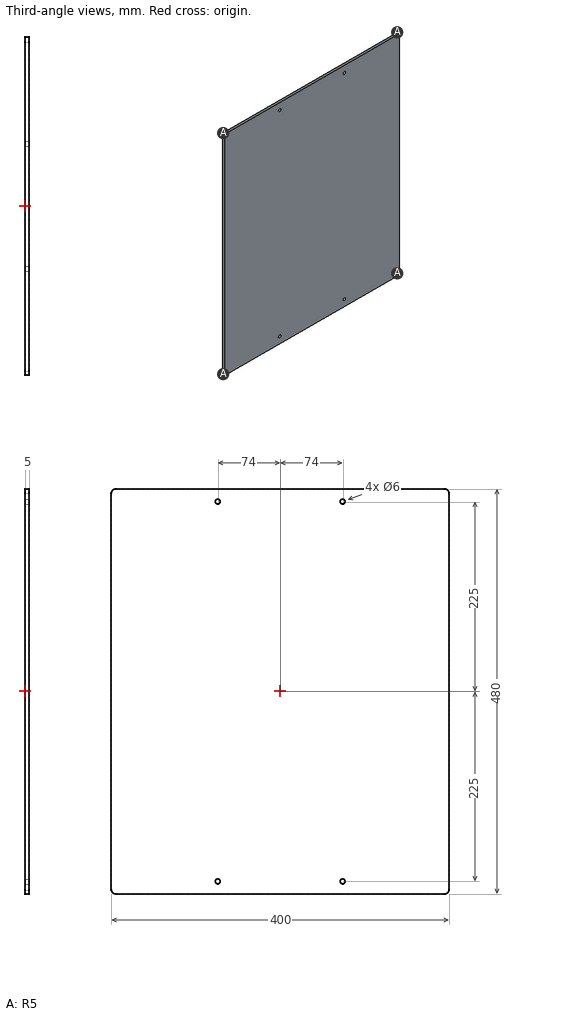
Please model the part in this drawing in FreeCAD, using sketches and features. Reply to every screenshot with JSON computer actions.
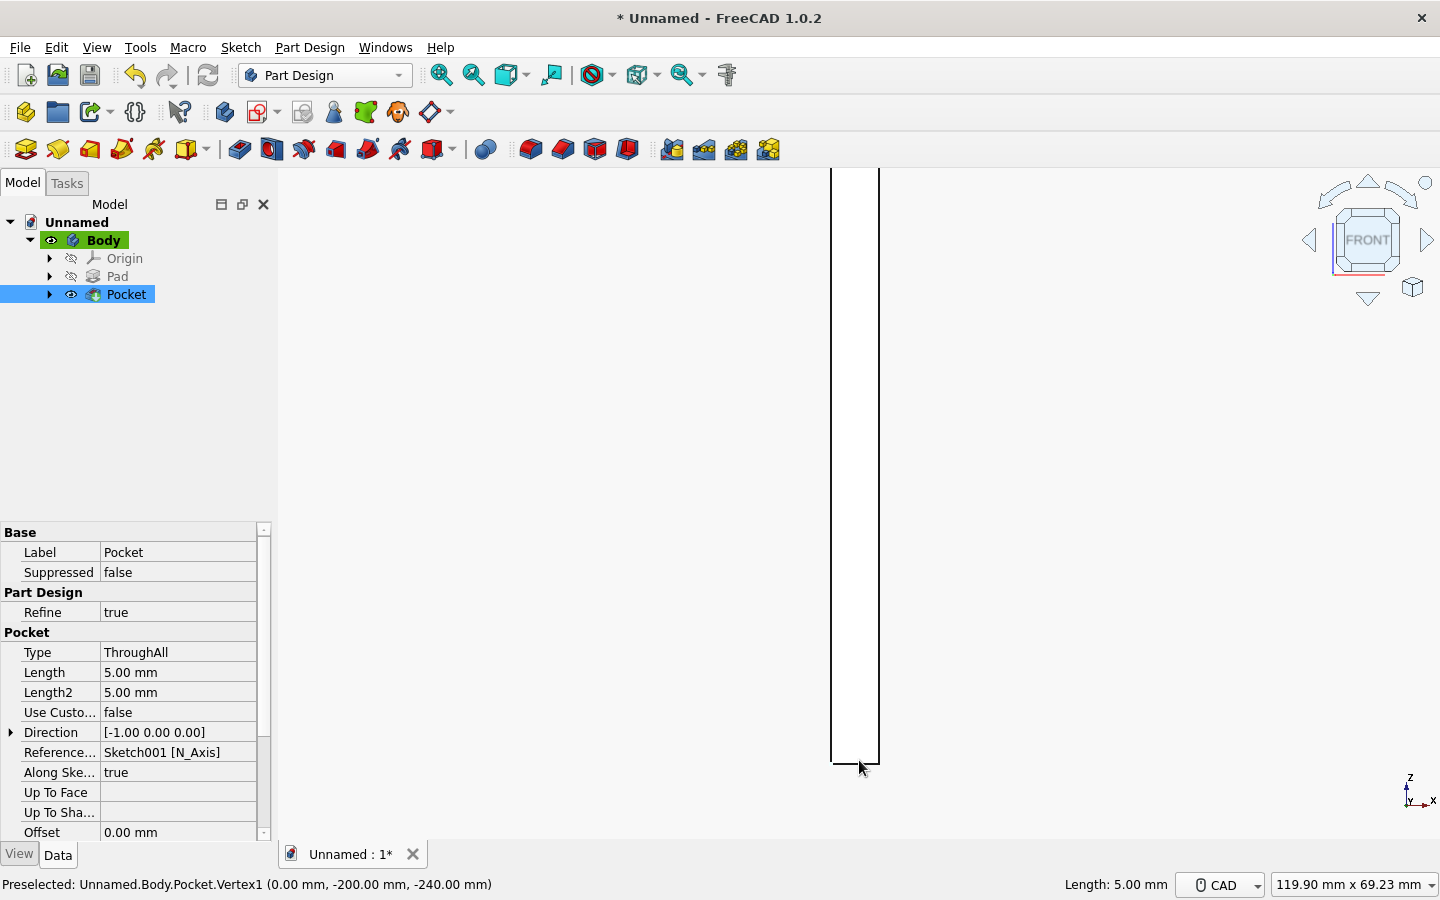
{"action": "left_click", "coordinate": [855, 763], "text": "ctrl"}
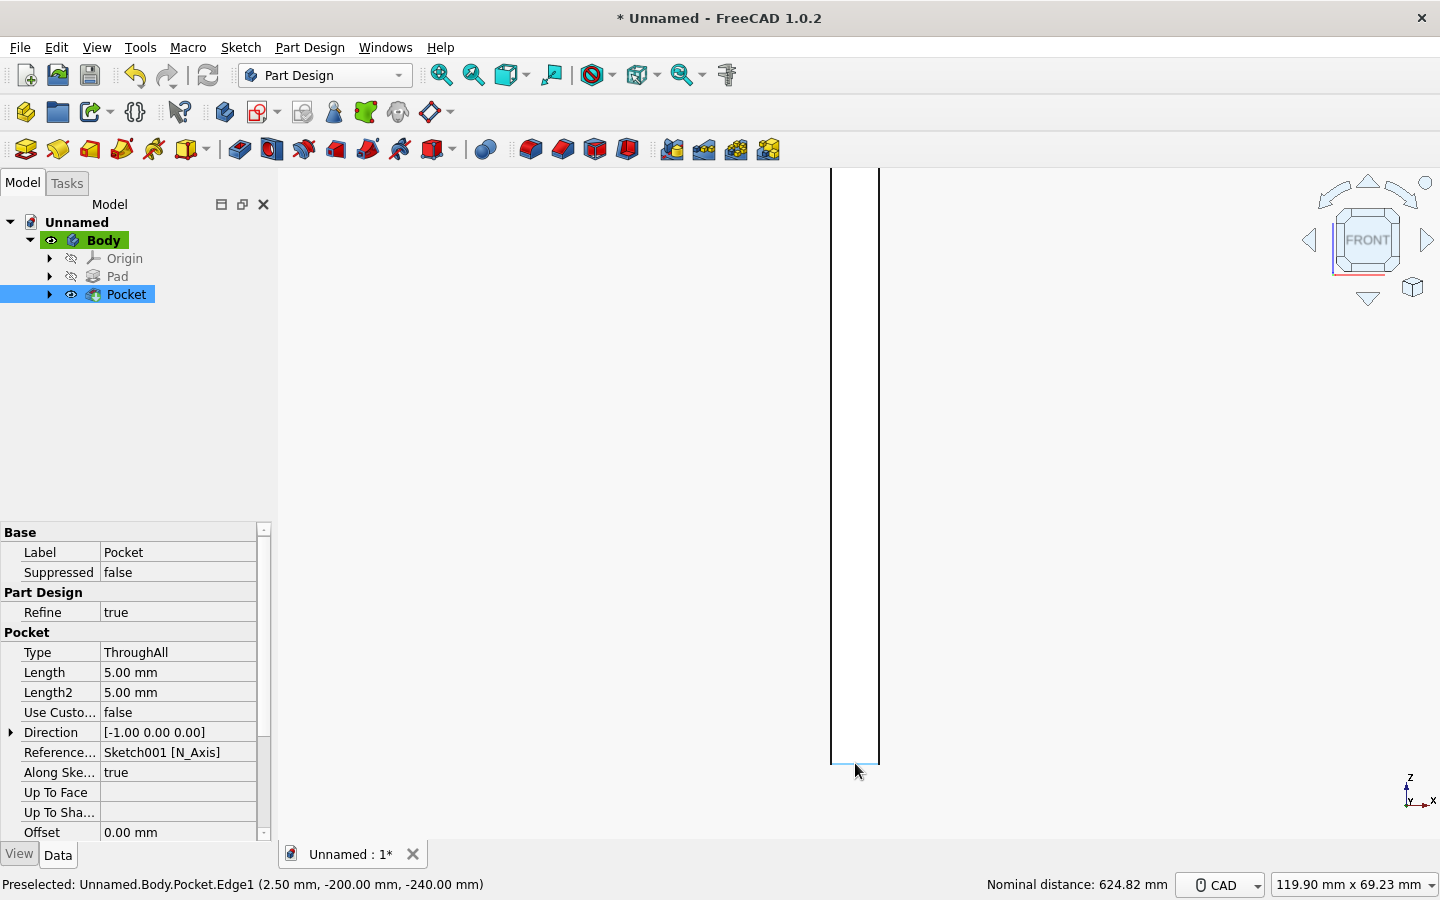
{"action": "left_click", "coordinate": [442, 76]}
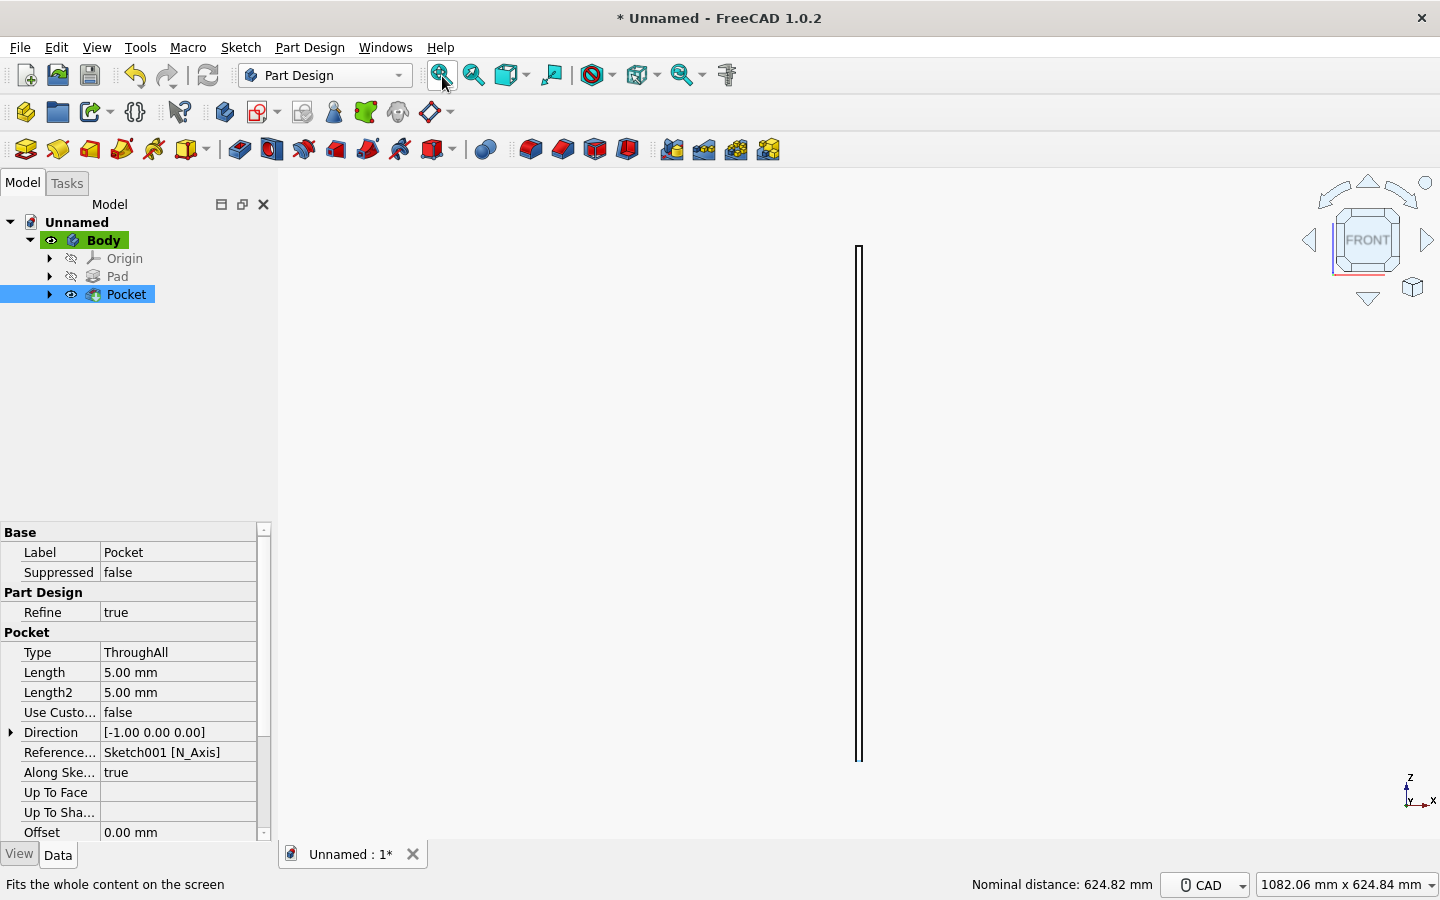
{"action": "key", "text": "3"}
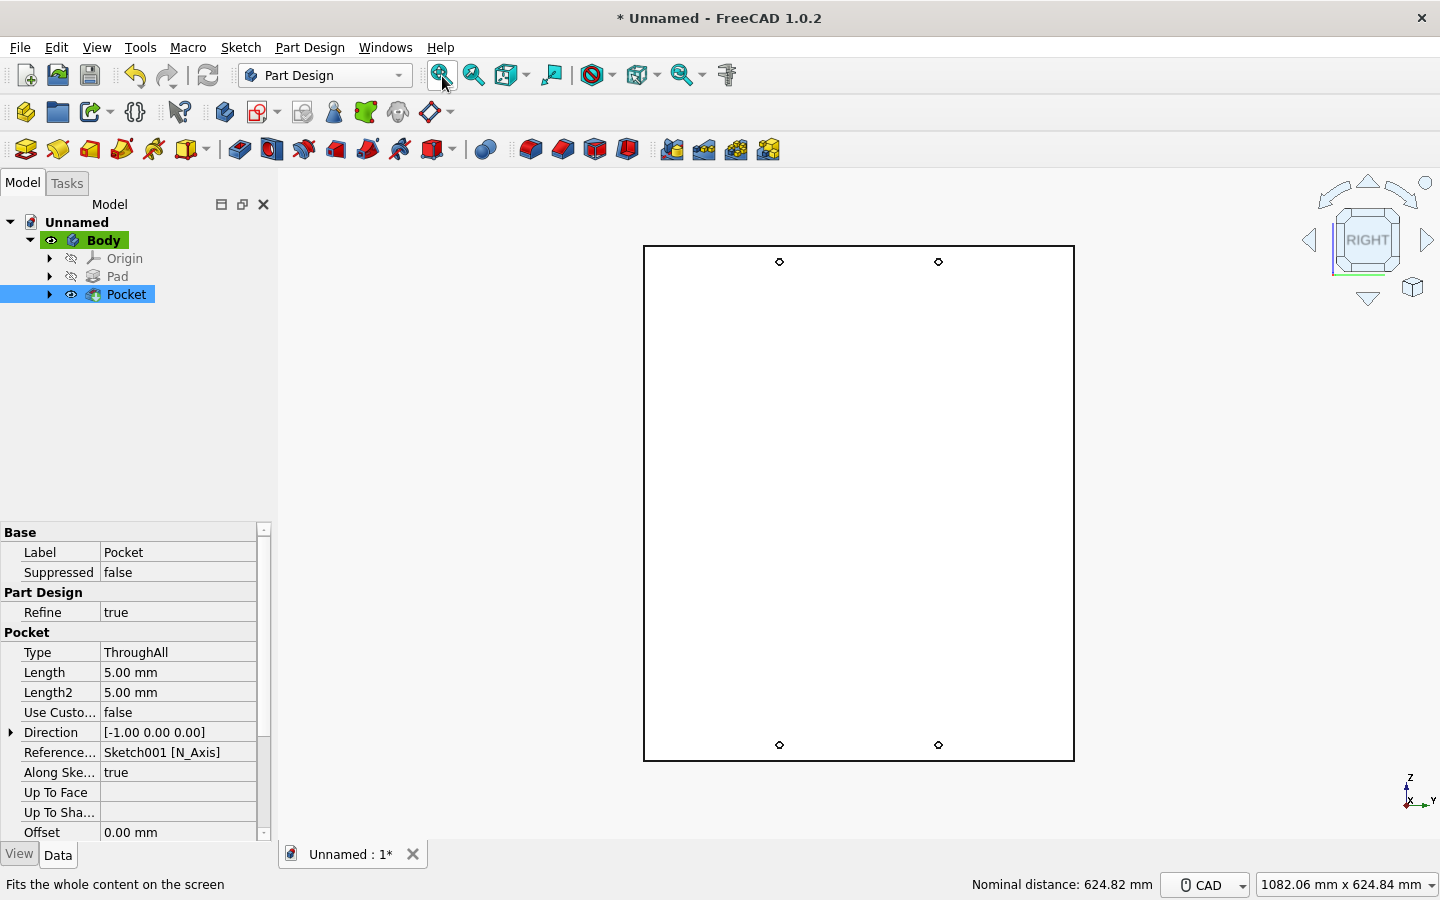
{"action": "scroll", "coordinate": [1074, 760], "scroll_direction": "up", "scroll_amount": 11}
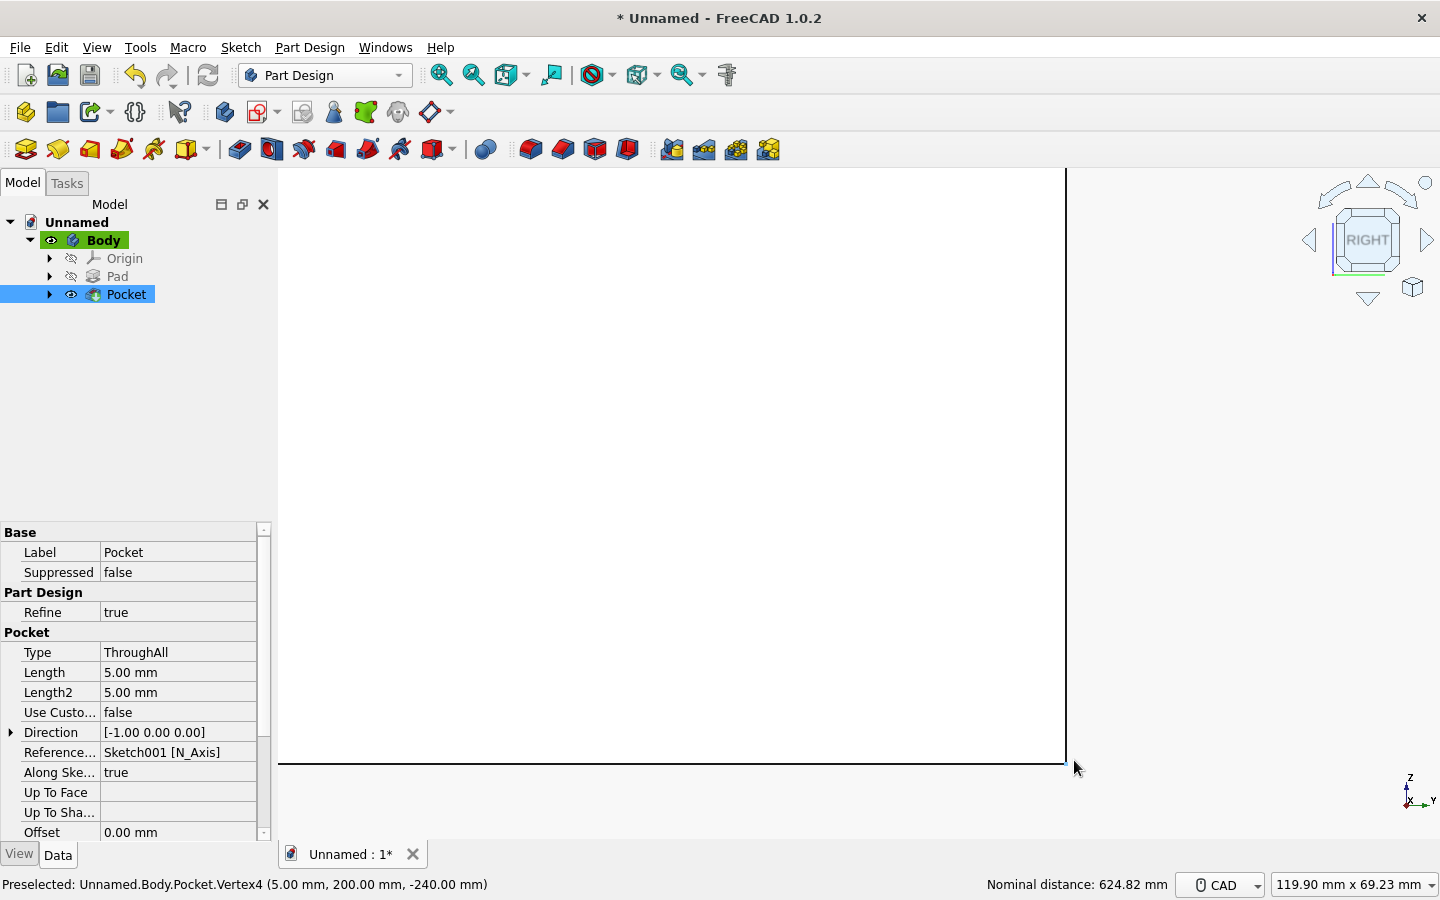
{"action": "key", "text": "v f"}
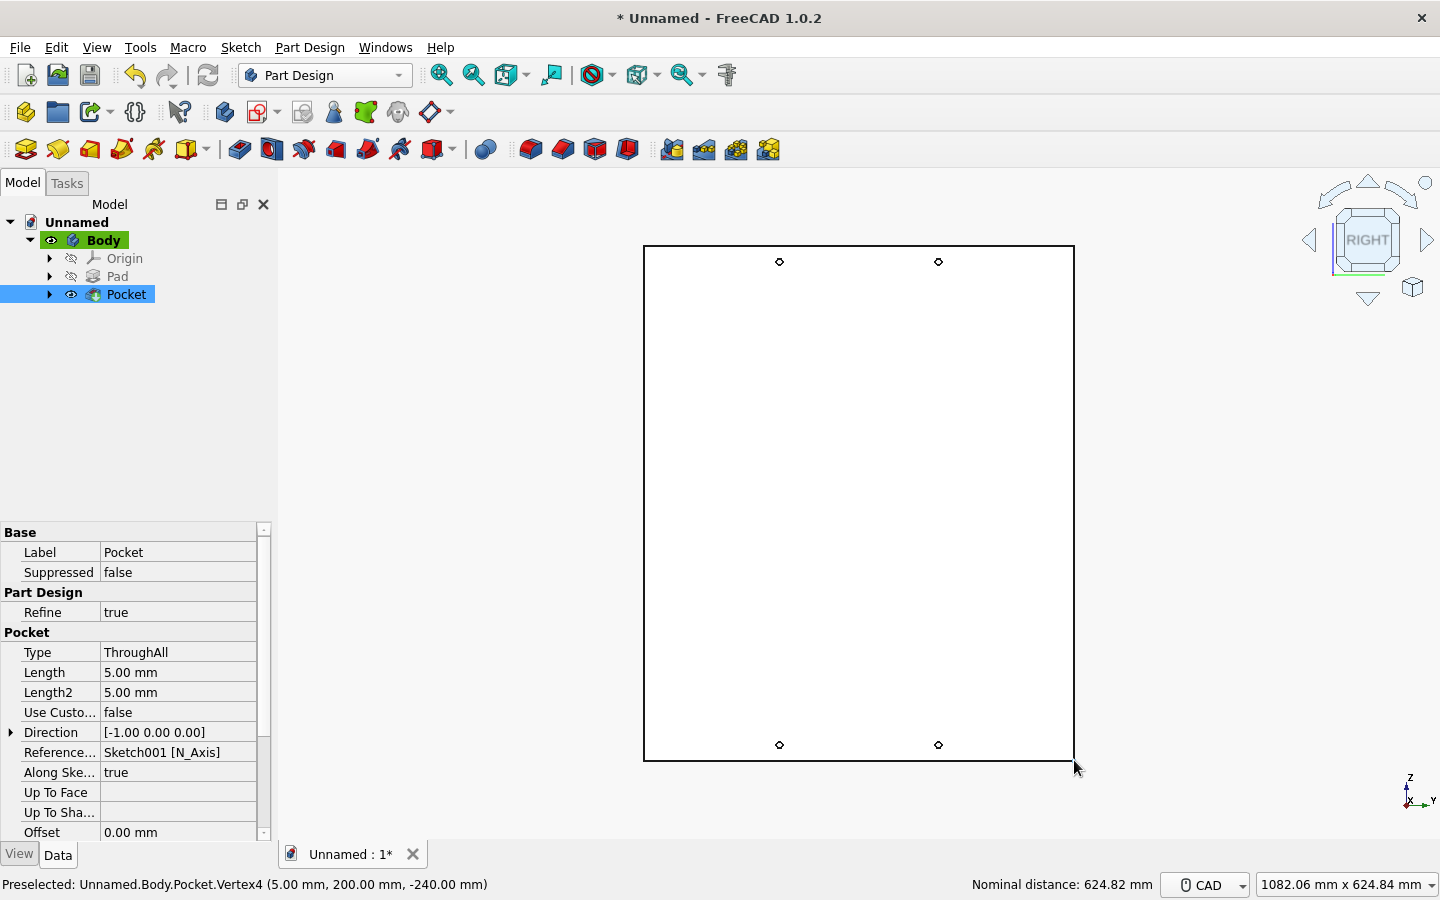
{"action": "key", "text": "5"}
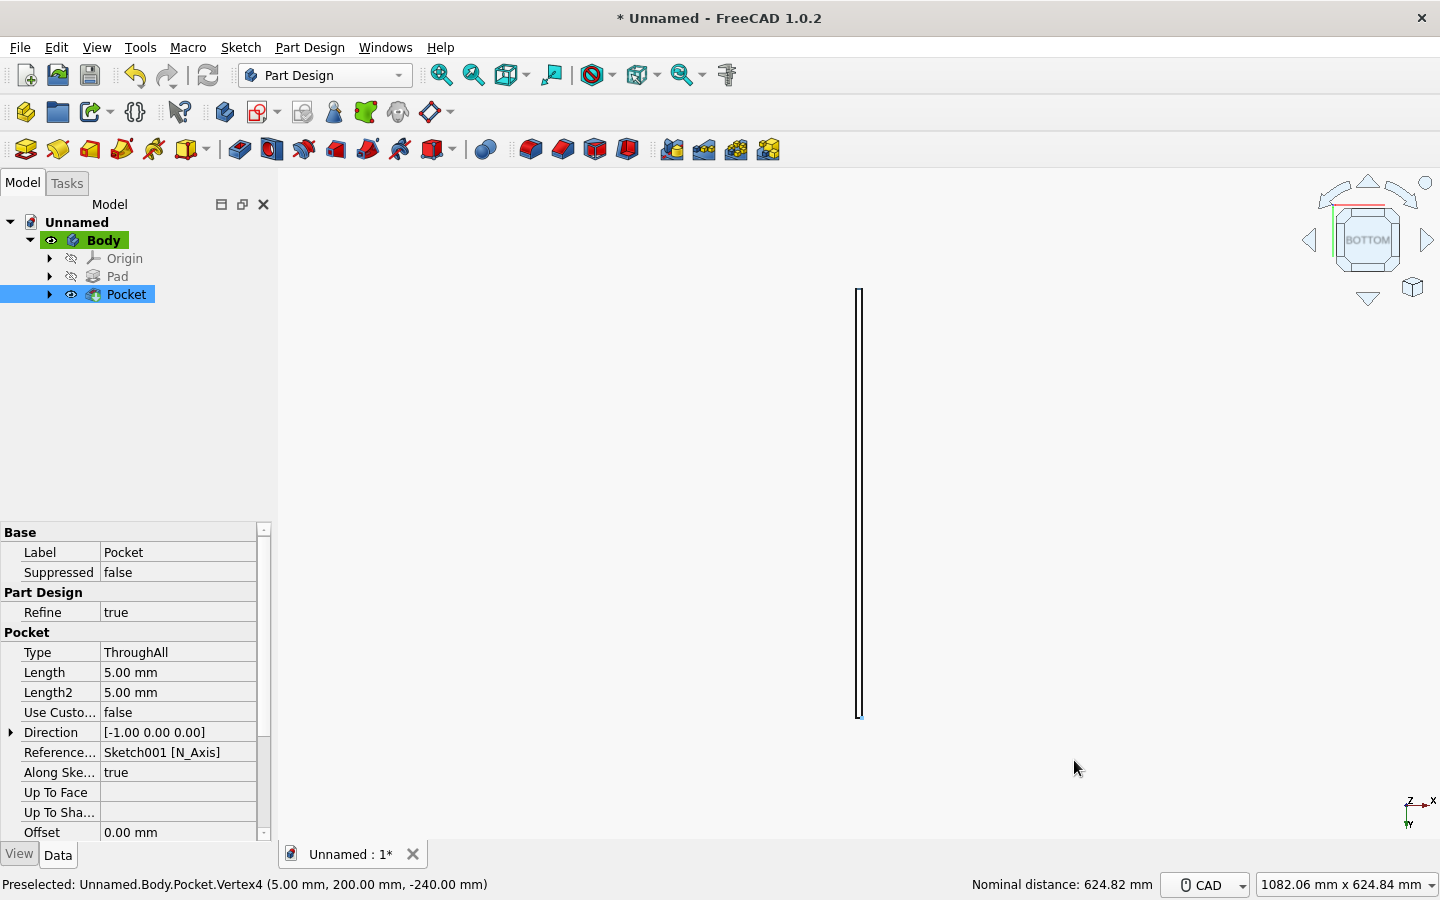
{"action": "scroll", "coordinate": [859, 717], "scroll_direction": "up", "scroll_amount": 11}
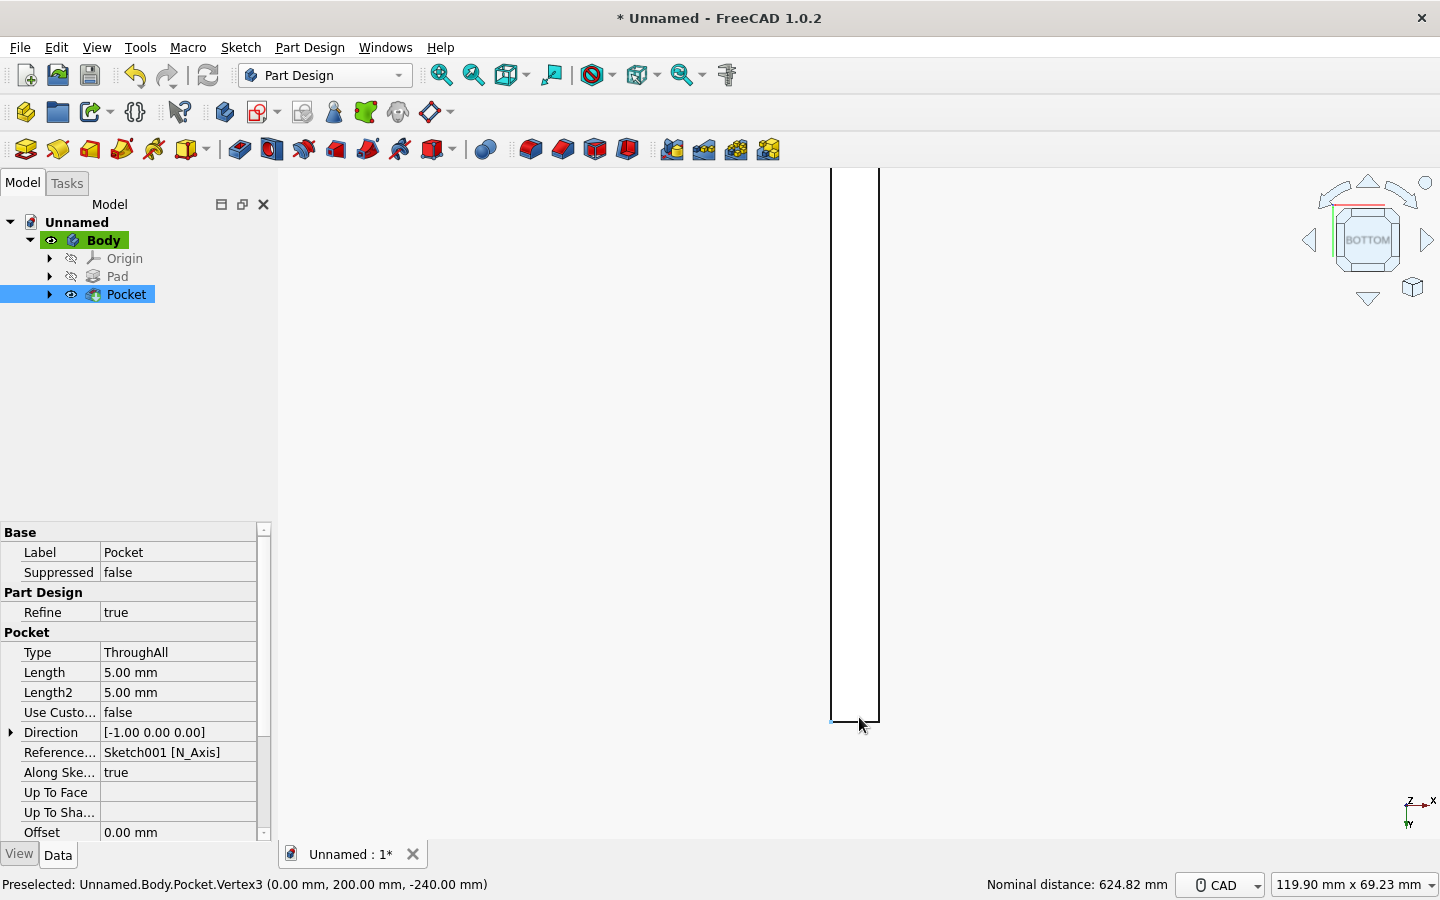
{"action": "left_click", "coordinate": [855, 721], "text": "ctrl"}